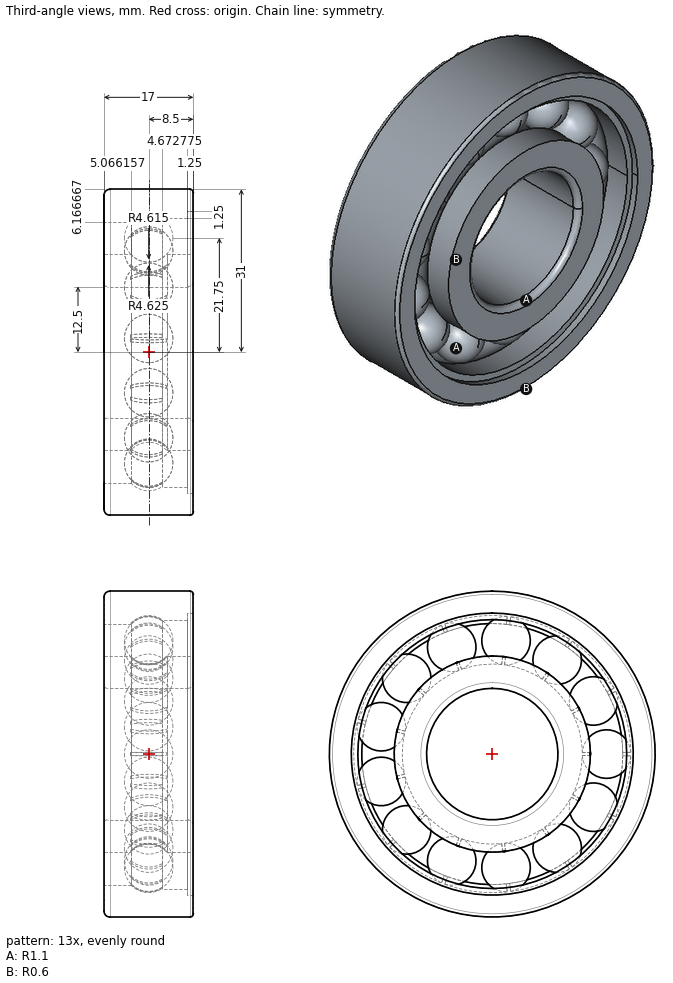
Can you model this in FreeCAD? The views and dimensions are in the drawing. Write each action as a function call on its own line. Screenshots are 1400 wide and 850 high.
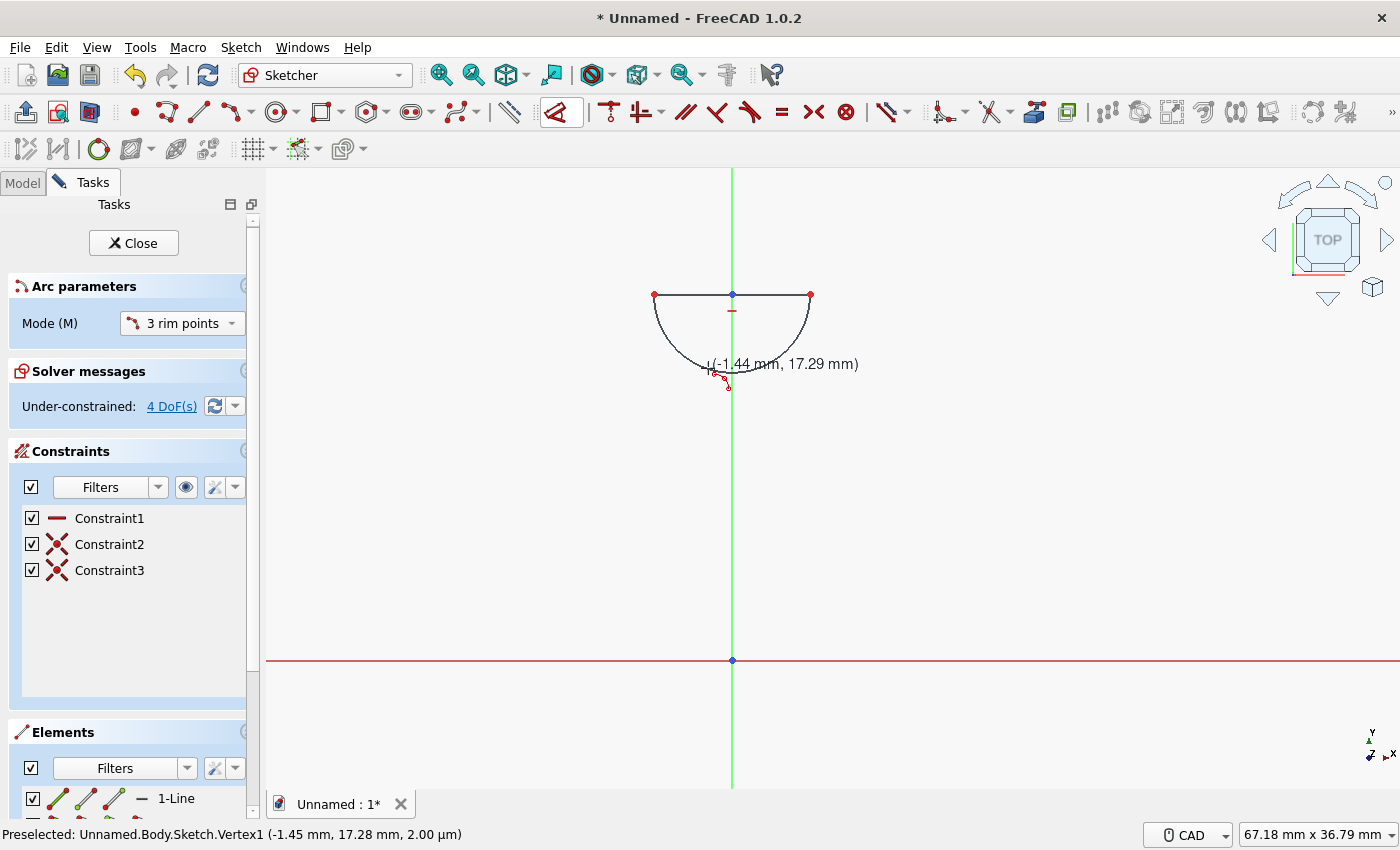
click(200, 112)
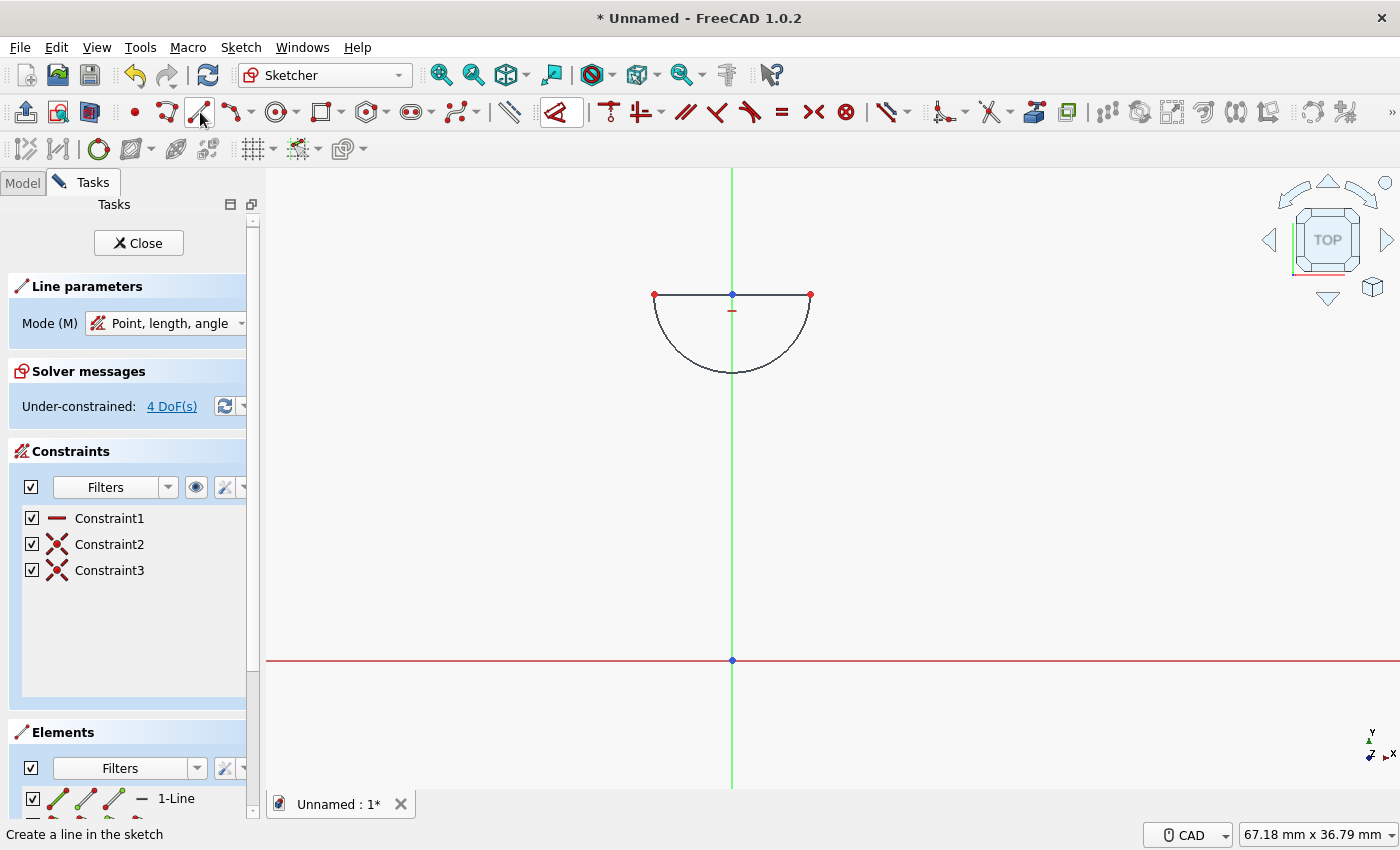
click(826, 294)
click(873, 294)
key(Escape)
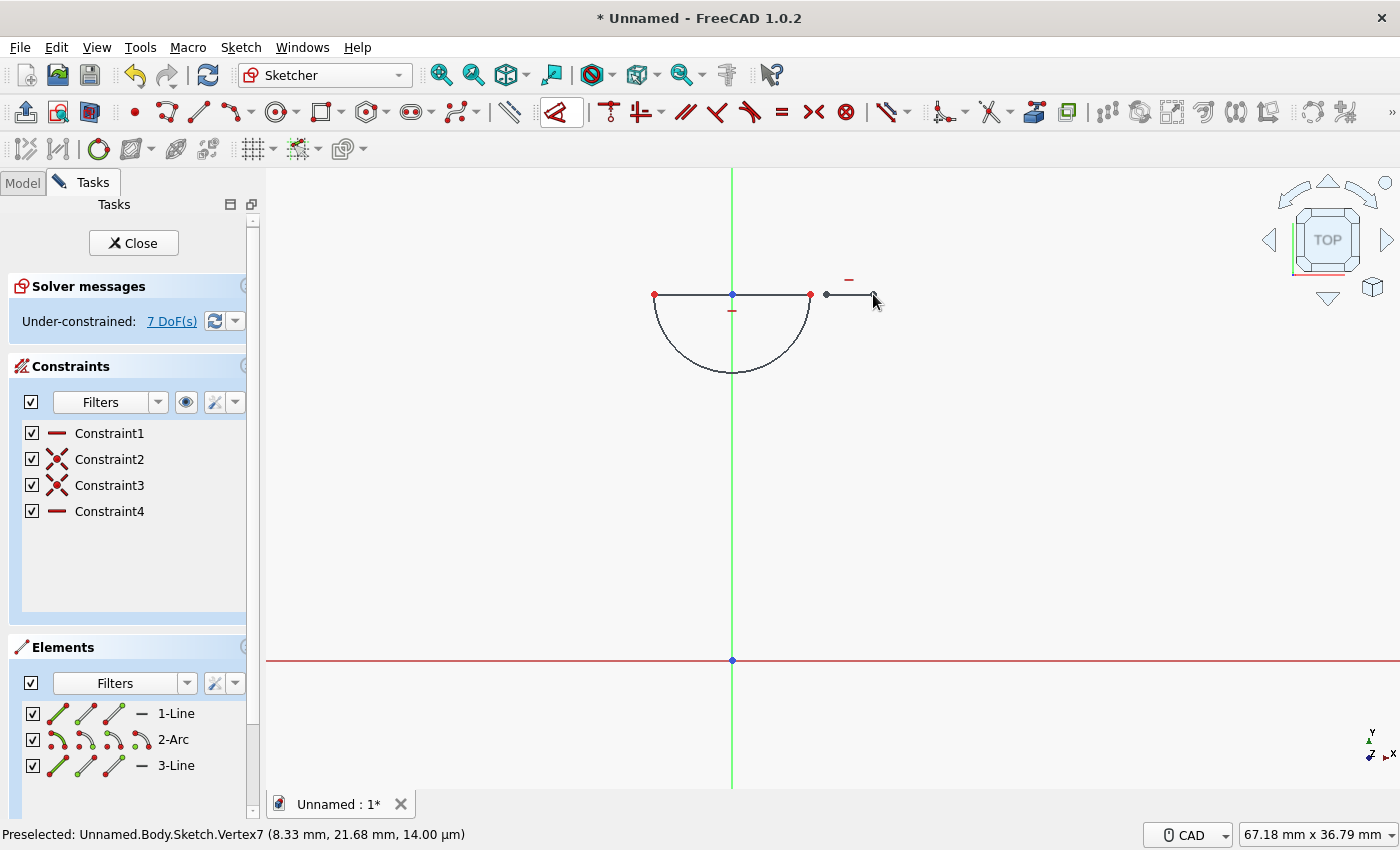
click(840, 295)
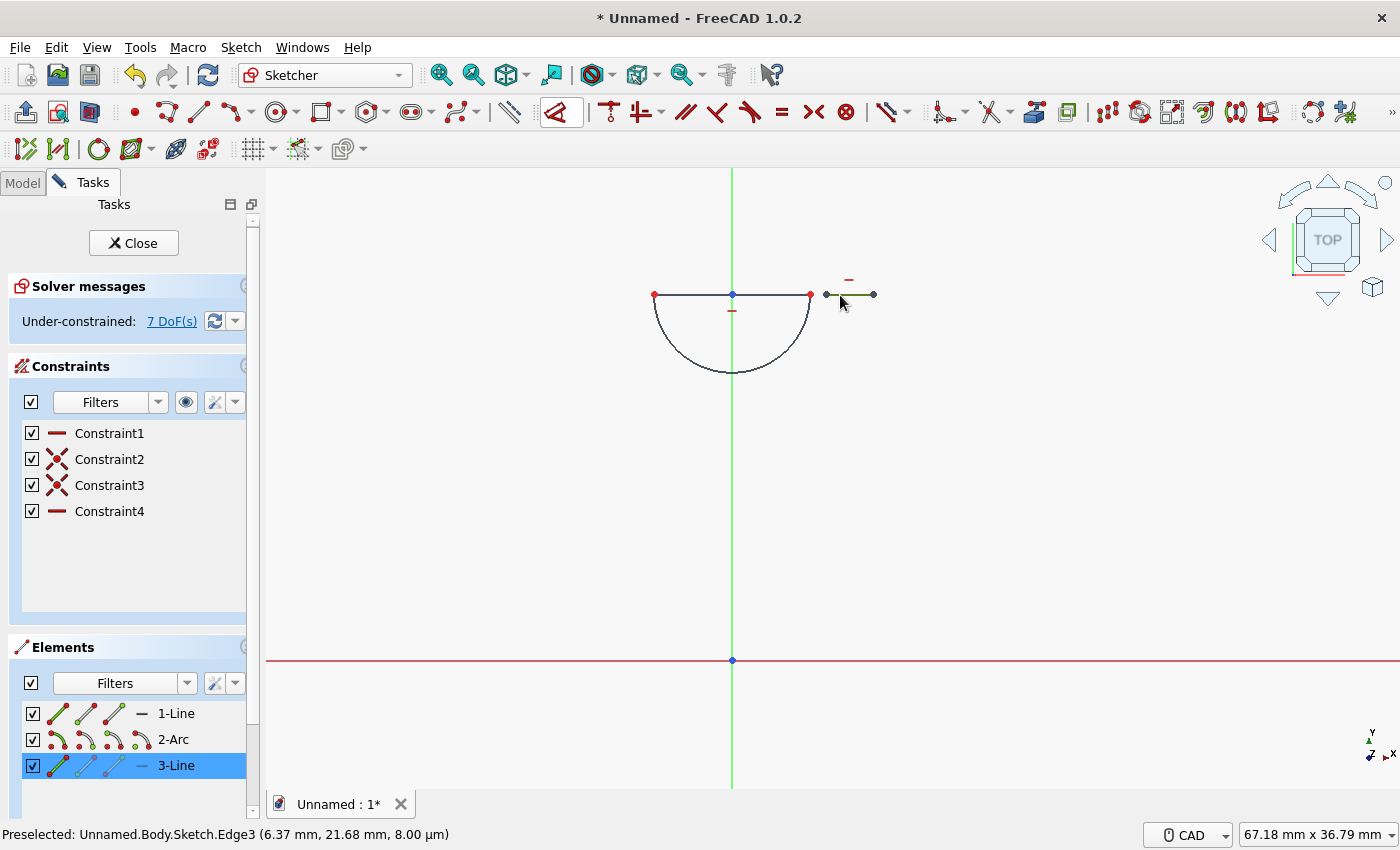
click(510, 112)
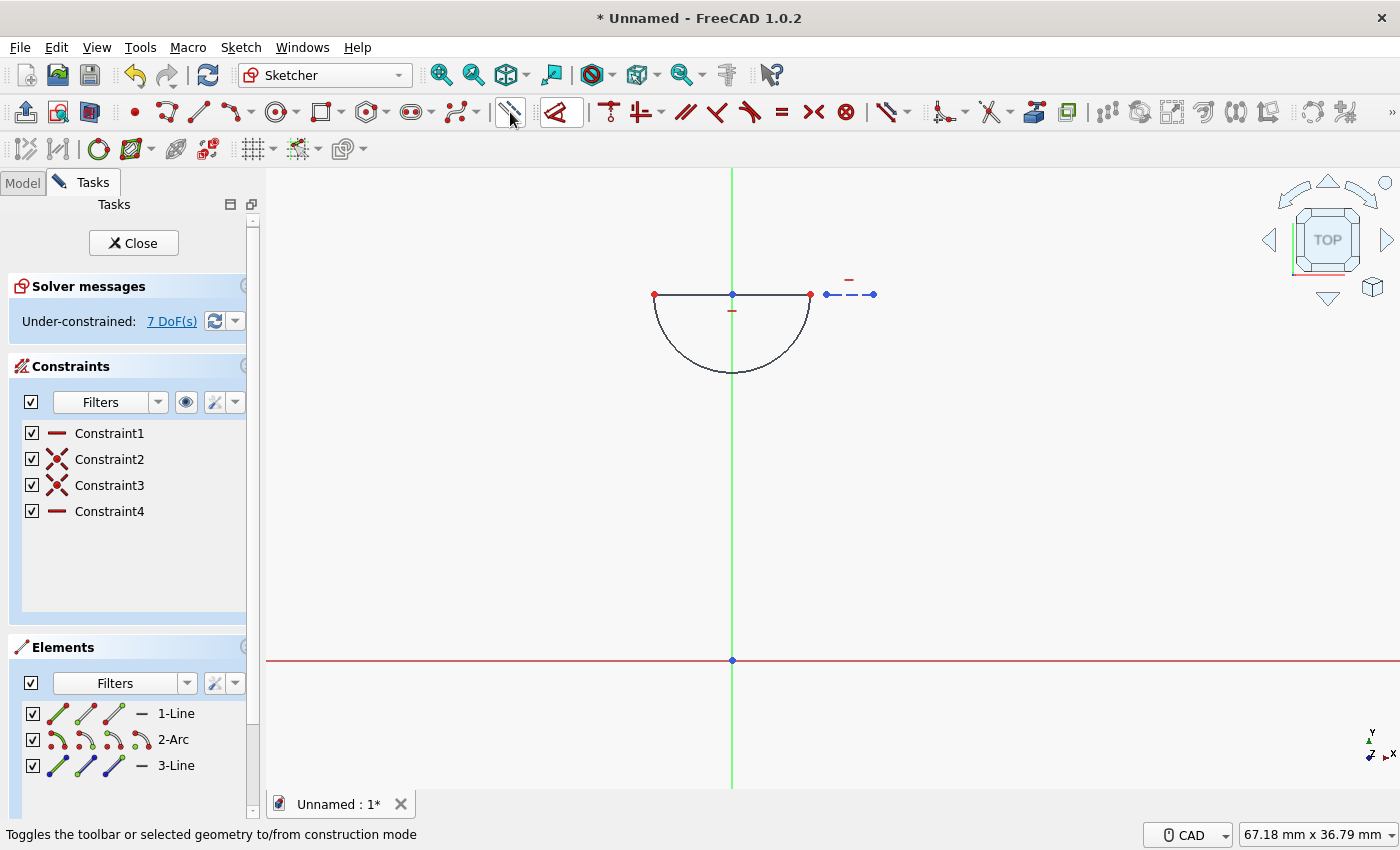
click(732, 295)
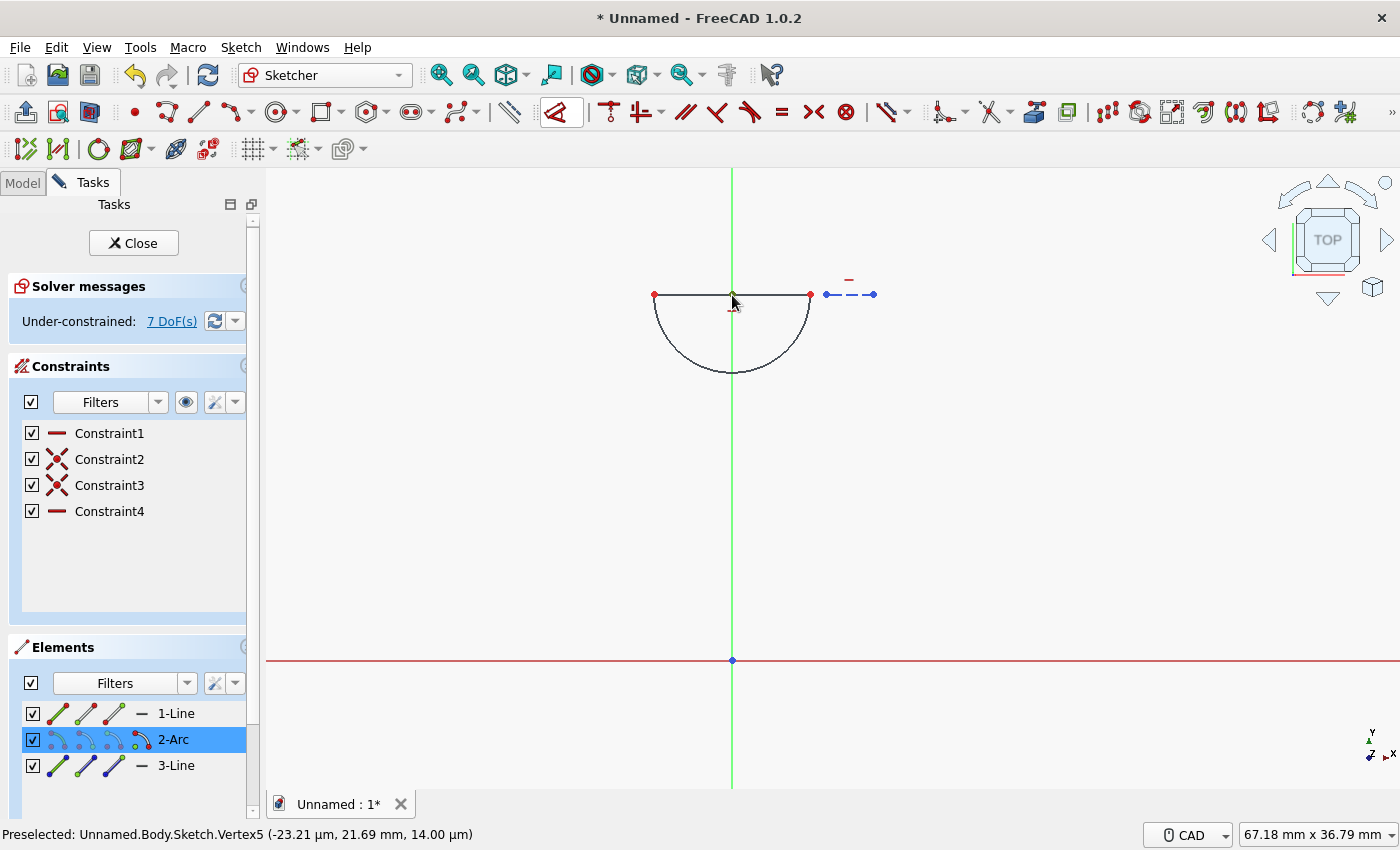
click(732, 721)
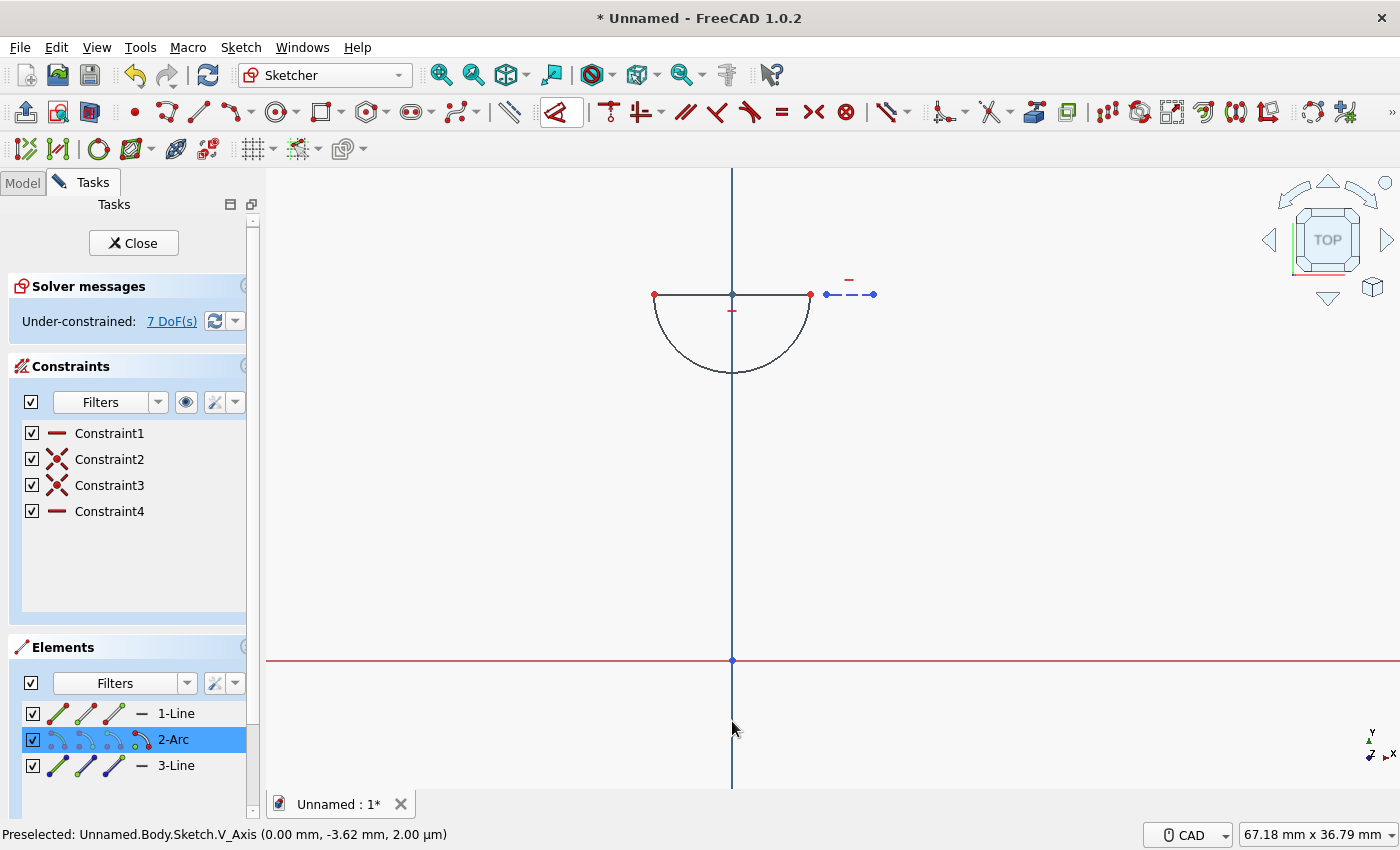
click(610, 112)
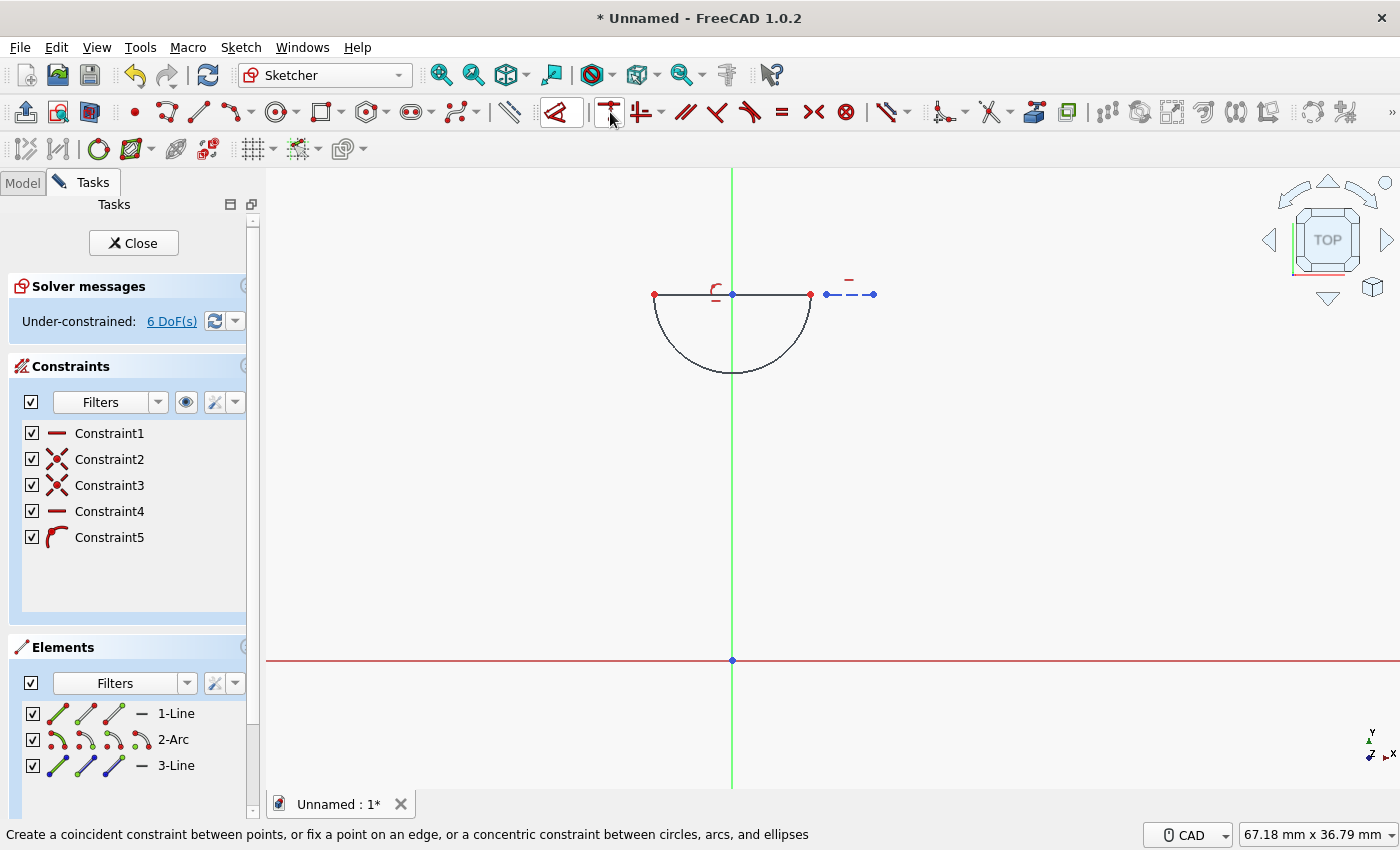
click(686, 358)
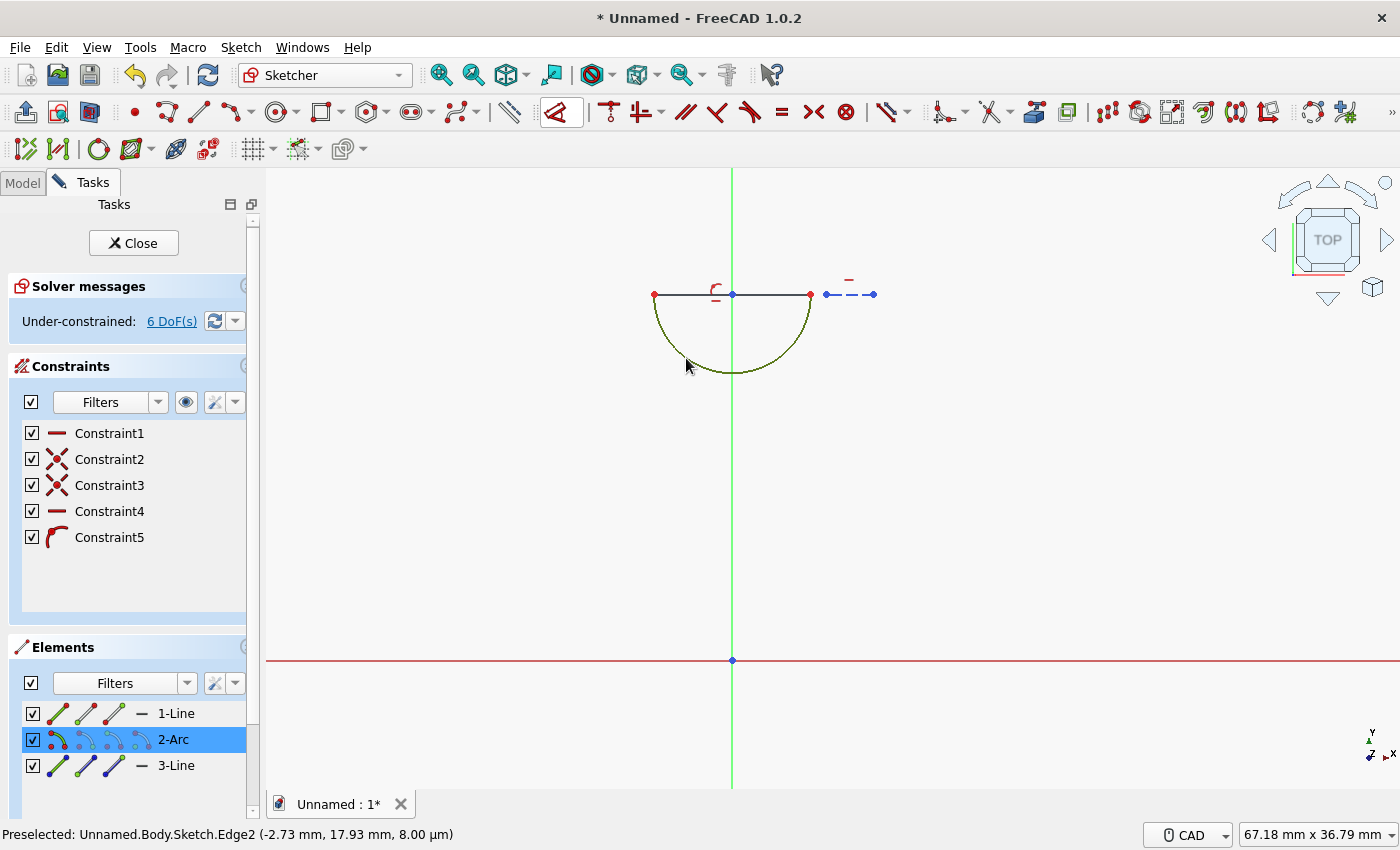
key(k)
key(r)